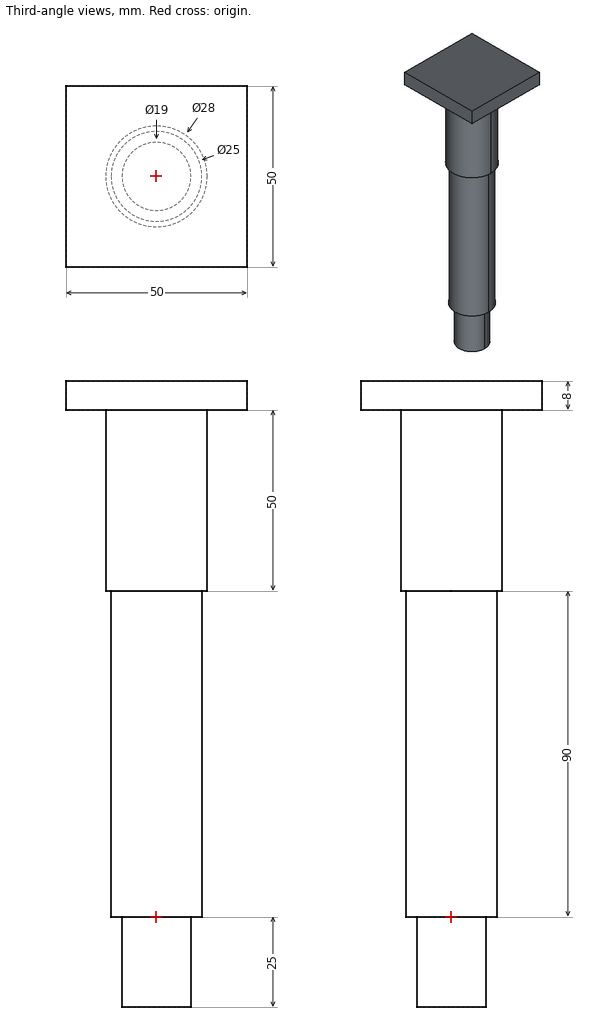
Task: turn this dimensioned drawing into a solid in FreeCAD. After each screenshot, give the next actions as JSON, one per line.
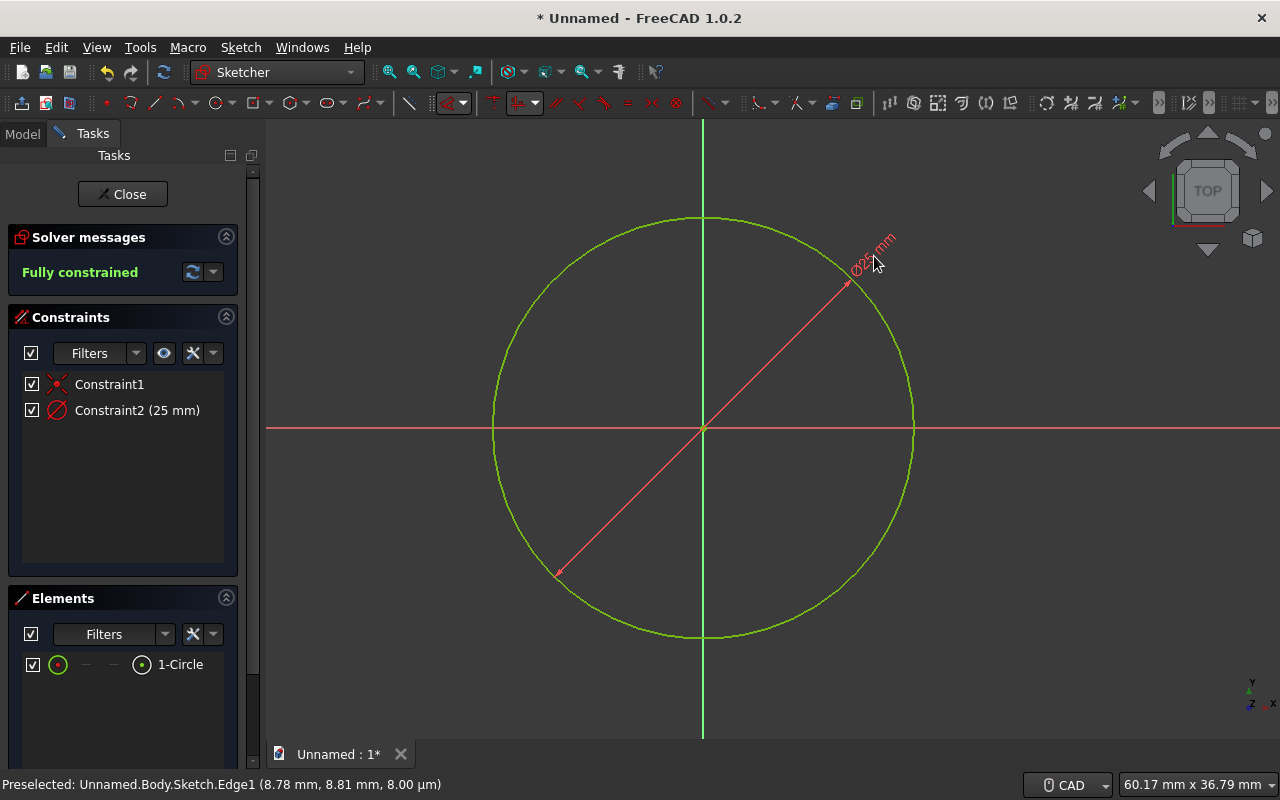
{"action": "left_click", "coordinate": [123, 194]}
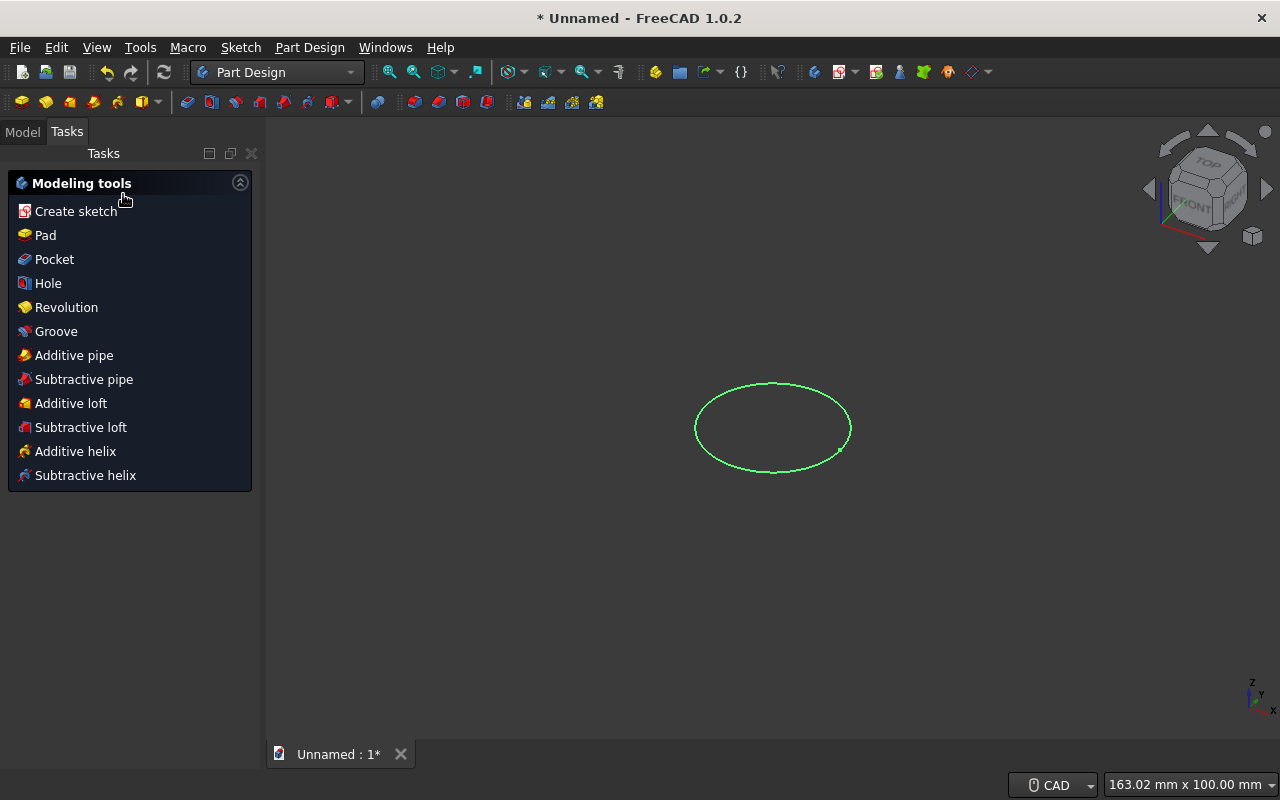
{"action": "left_click", "coordinate": [22, 102]}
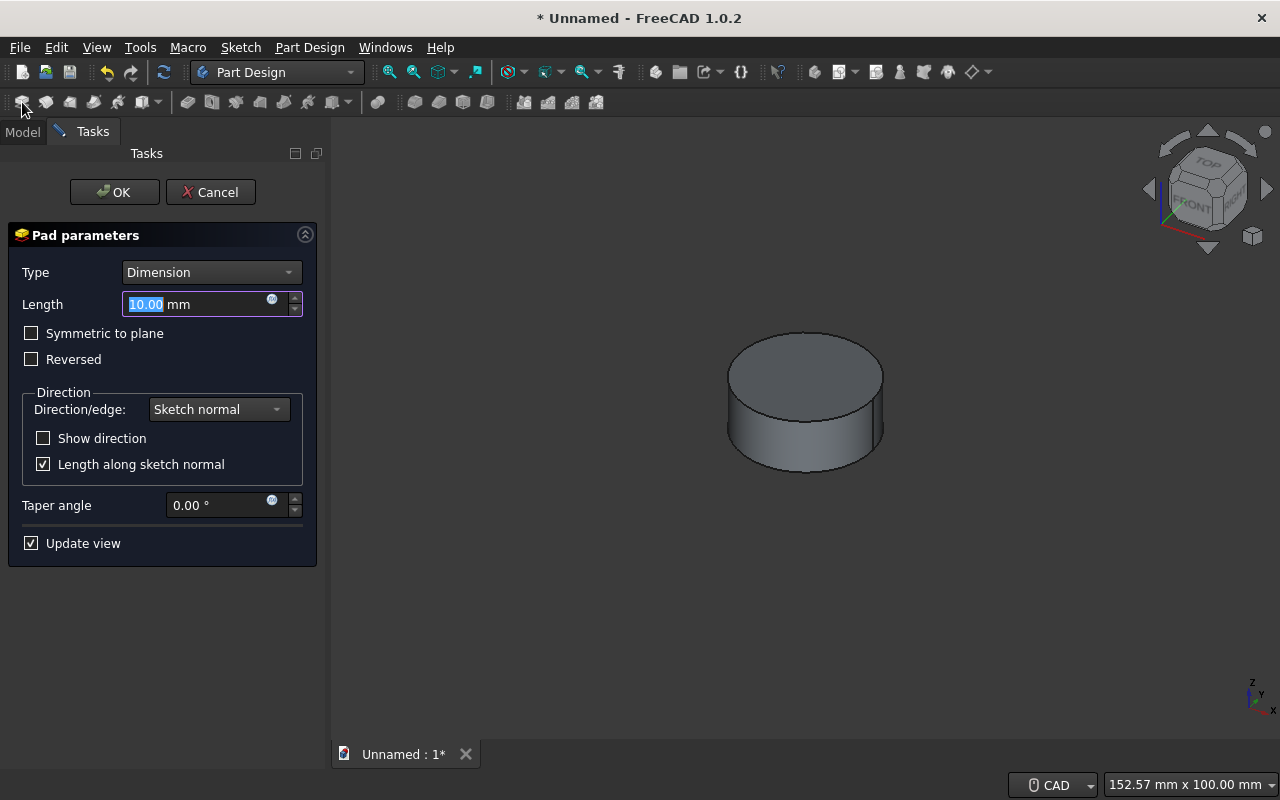
{"action": "type", "text": "90"}
{"action": "key", "text": "Tab"}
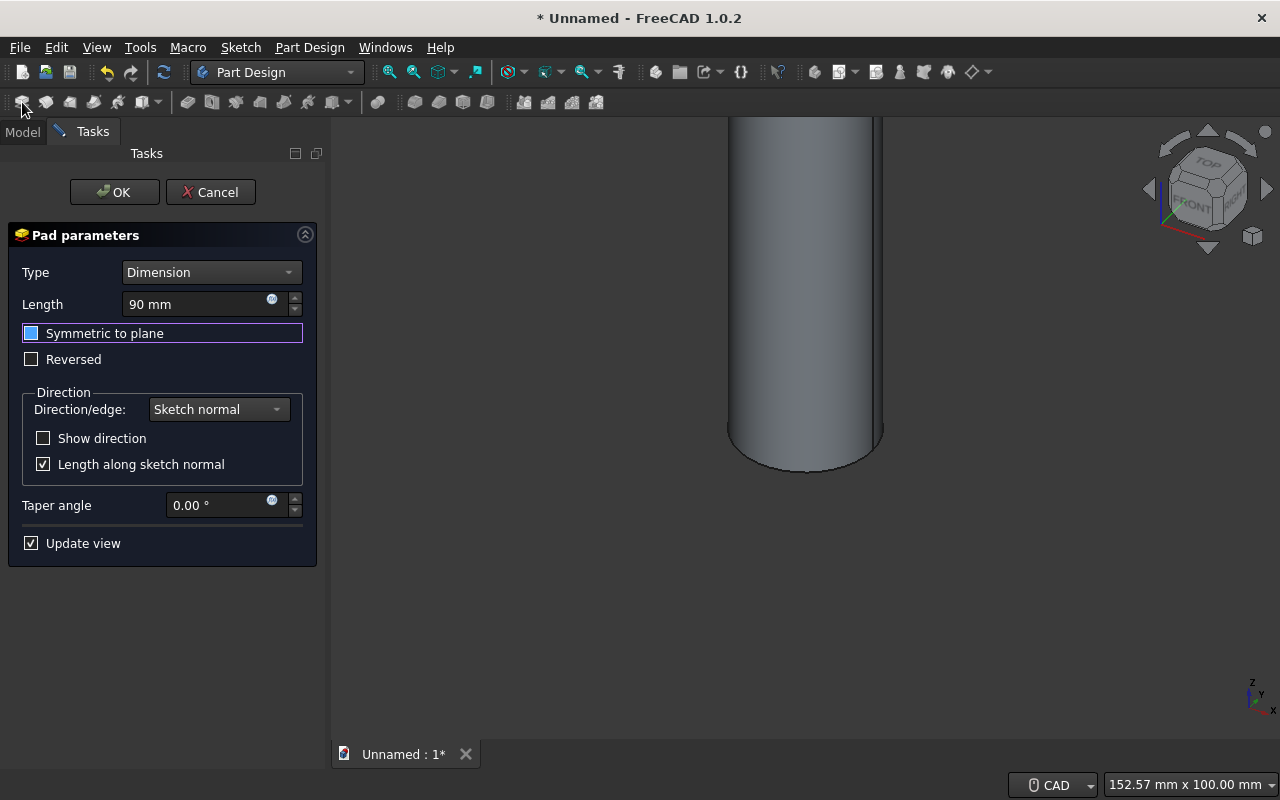
{"action": "left_click", "coordinate": [115, 192]}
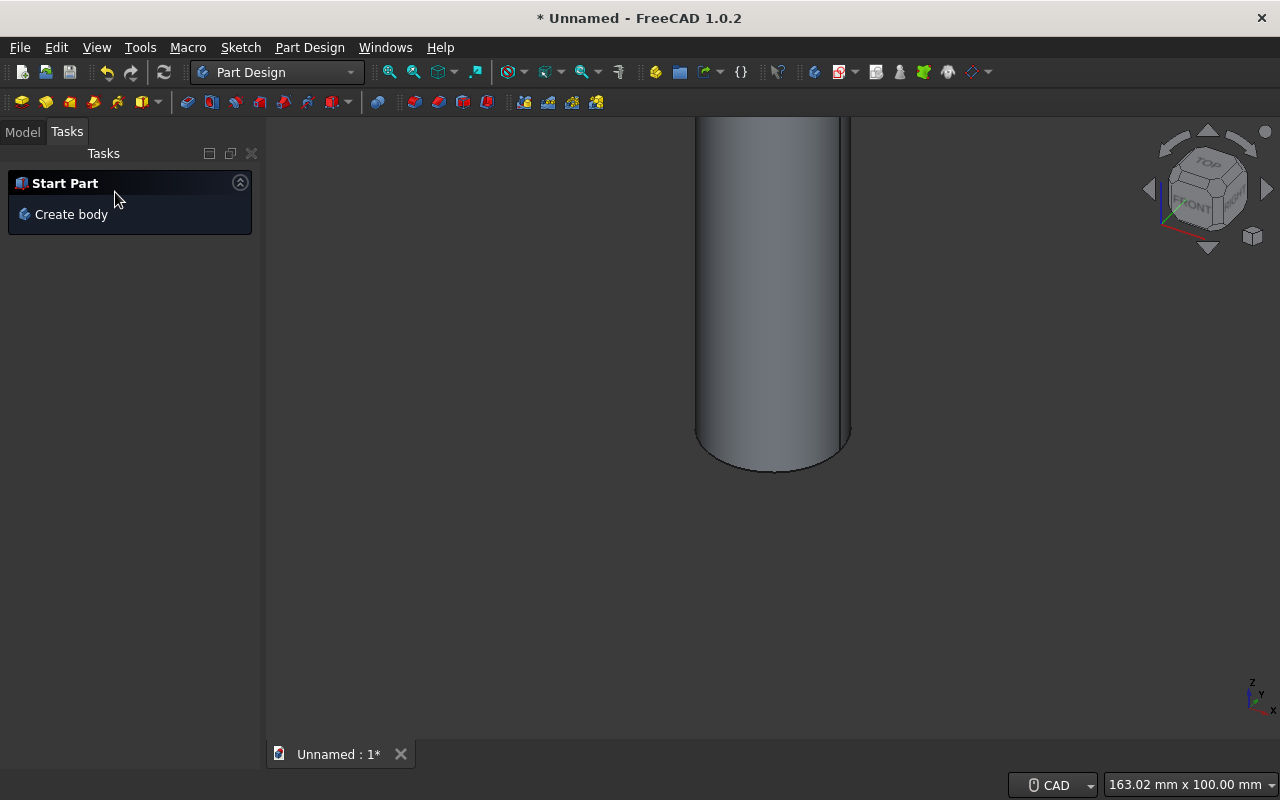
{"action": "key", "text": "v f"}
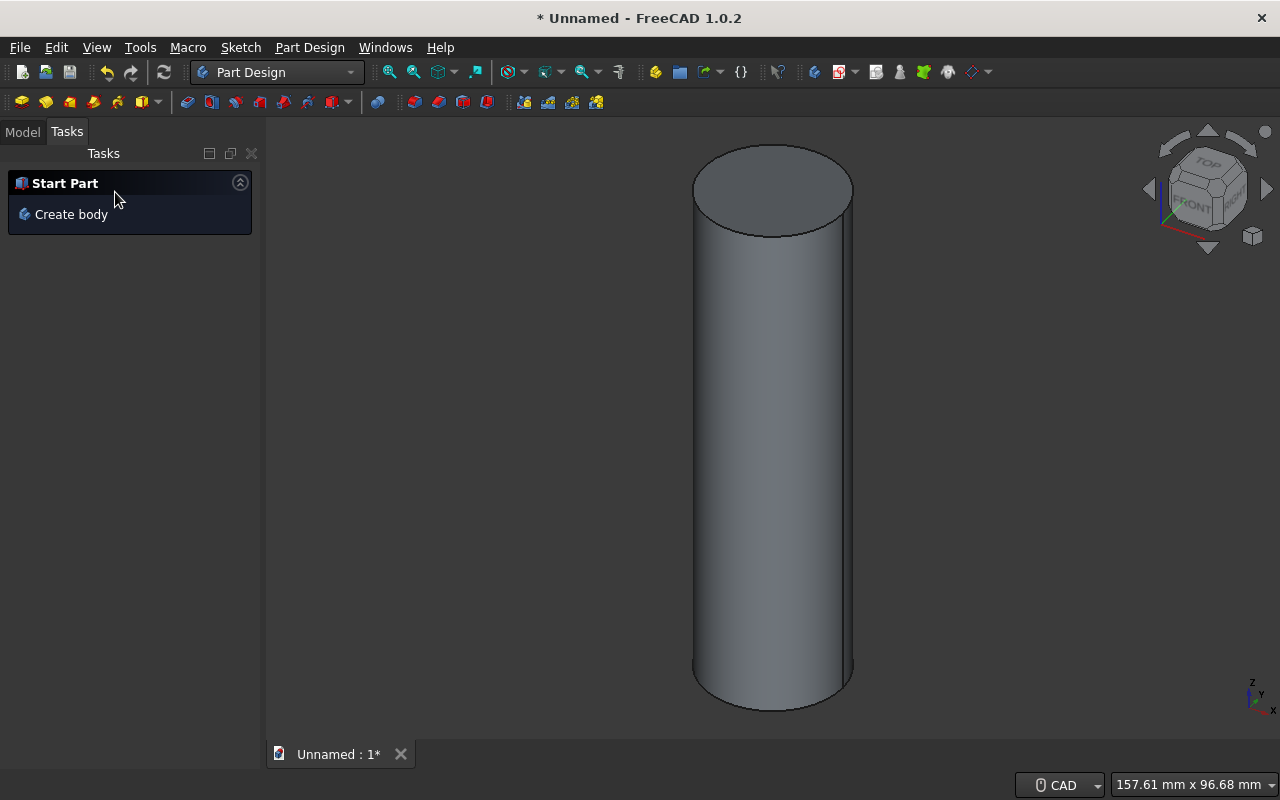
{"action": "left_click", "coordinate": [773, 190]}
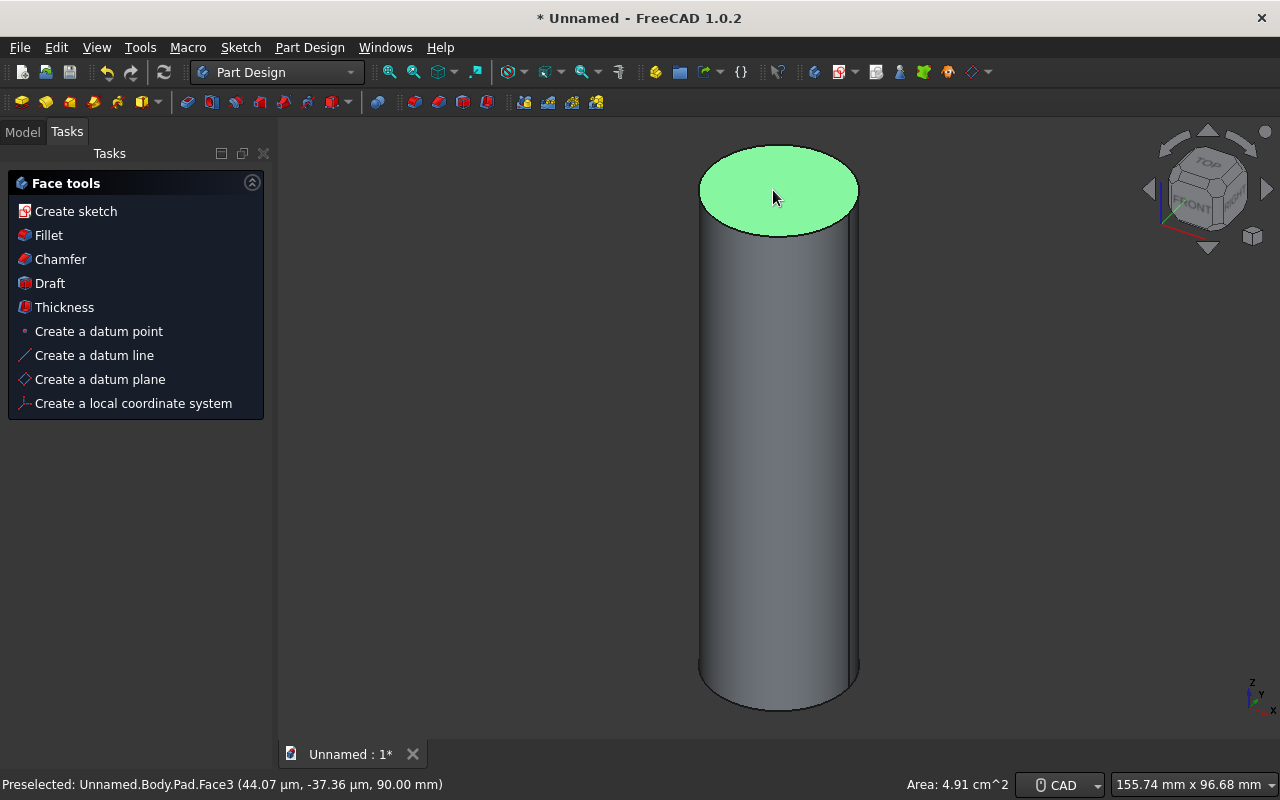
{"action": "left_click", "coordinate": [840, 72]}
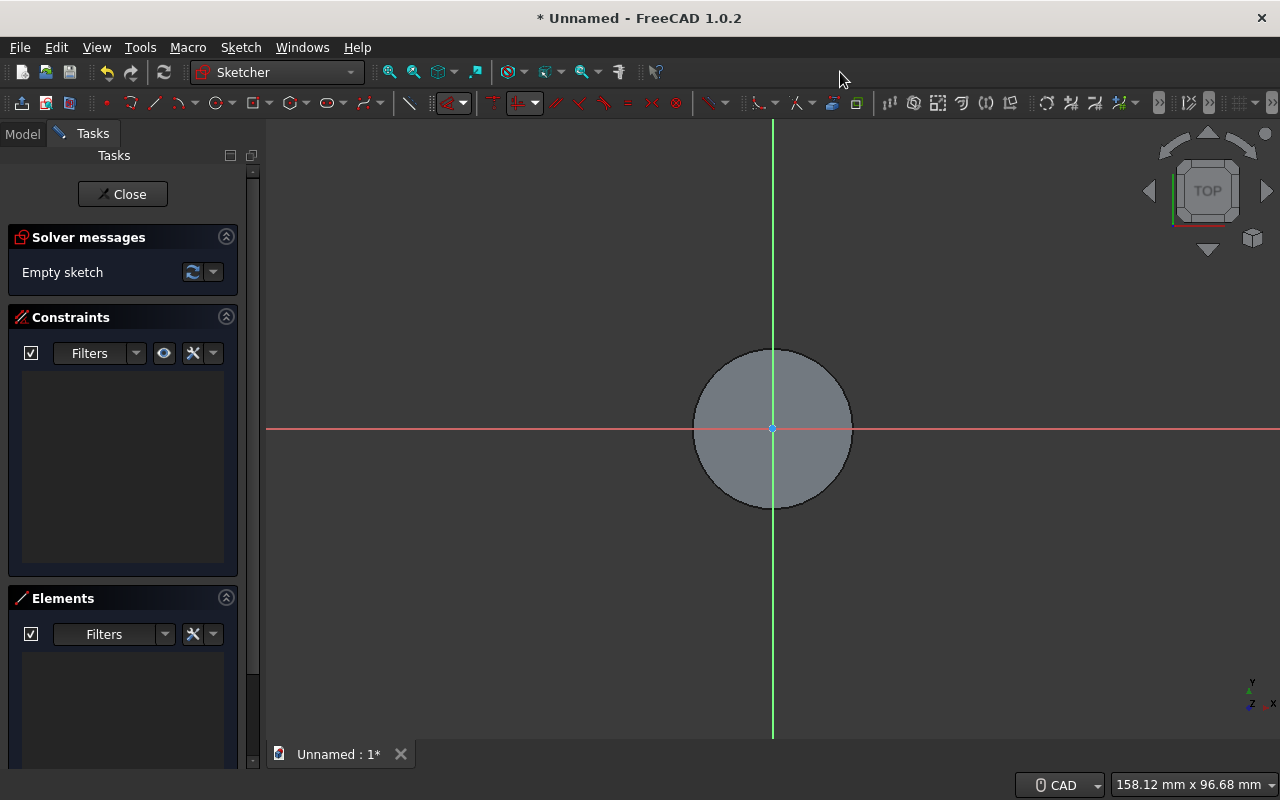
{"action": "scroll", "coordinate": [829, 429], "scroll_direction": "up", "scroll_amount": 4}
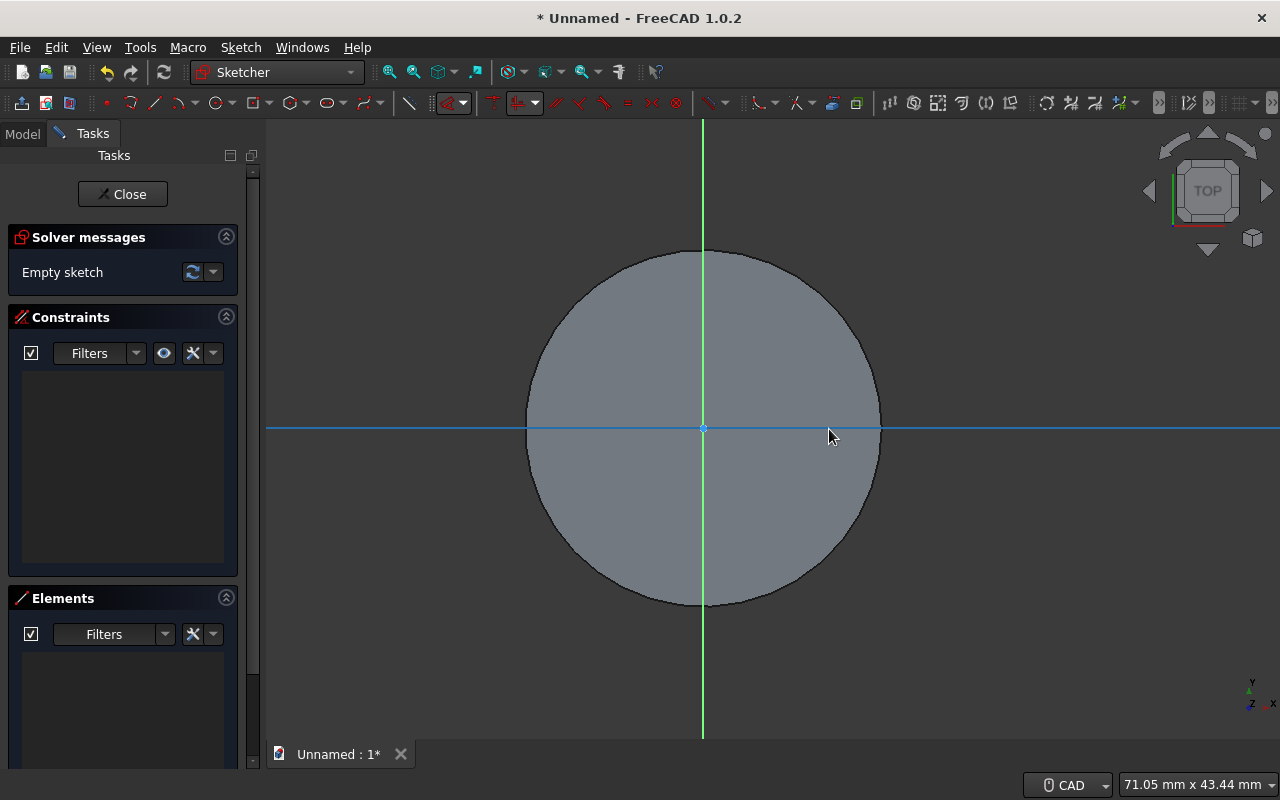
{"action": "key", "text": "g c"}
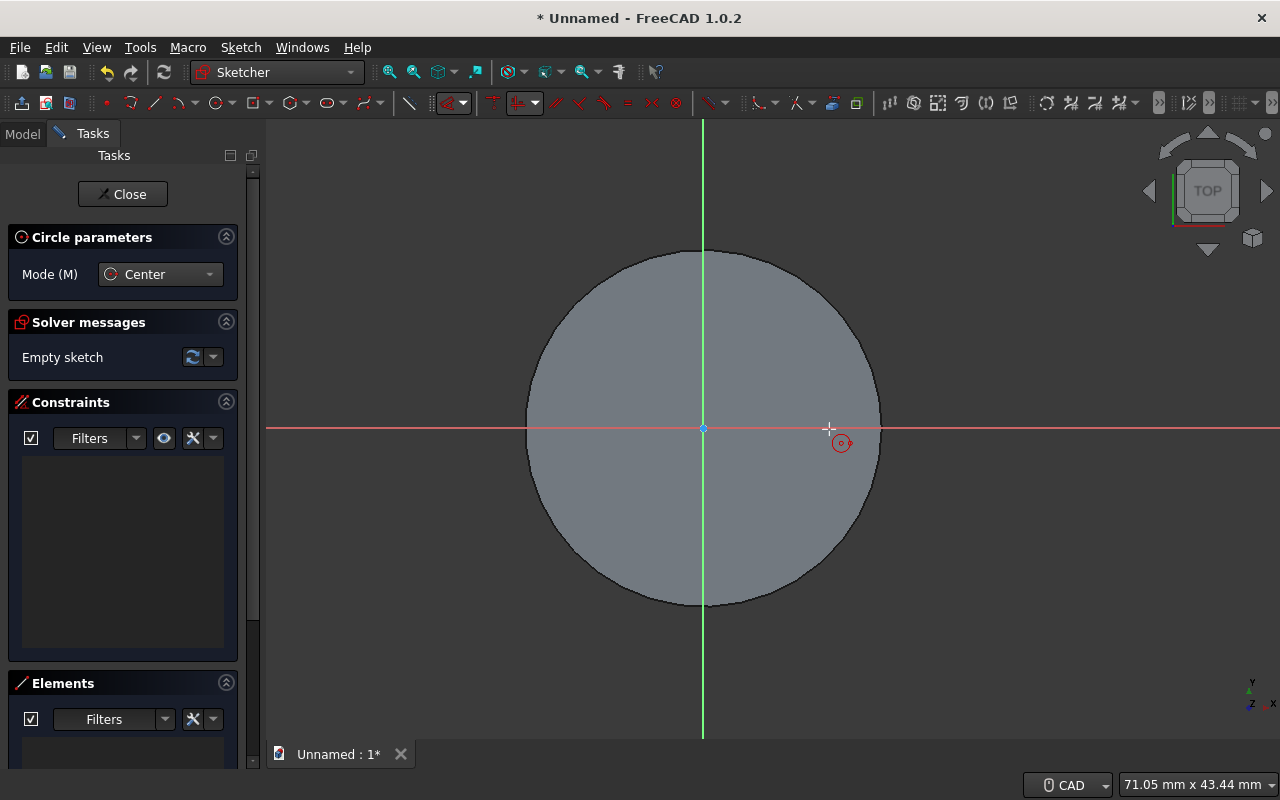
{"action": "left_click", "coordinate": [703, 428]}
{"action": "left_click", "coordinate": [845, 287]}
{"action": "key", "text": "Escape"}